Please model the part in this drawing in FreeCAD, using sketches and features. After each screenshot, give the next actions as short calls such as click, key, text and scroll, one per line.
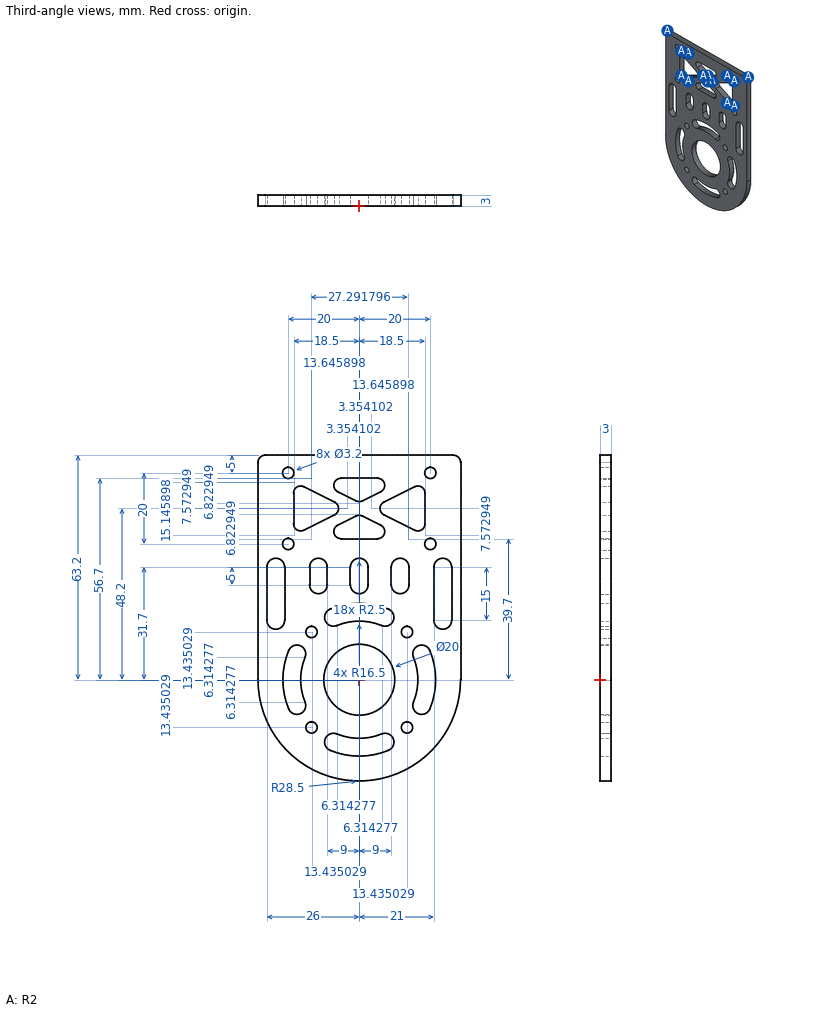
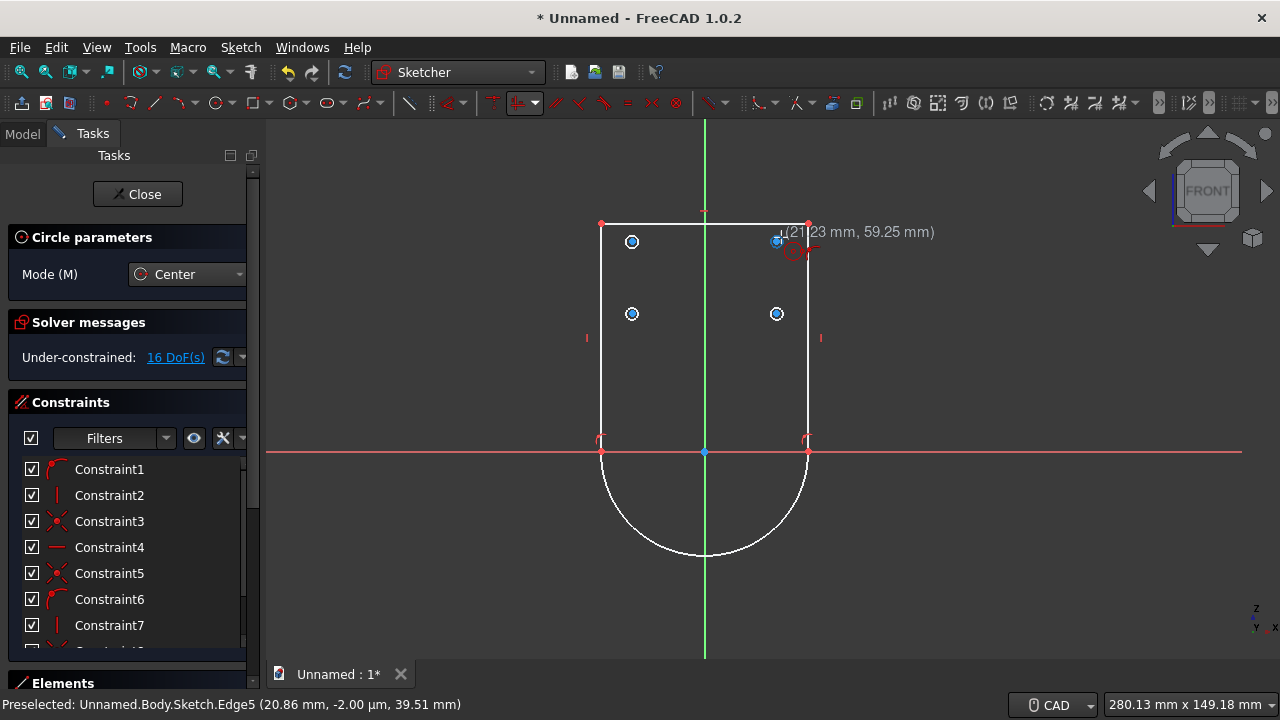
scroll(656, 403, up, 7)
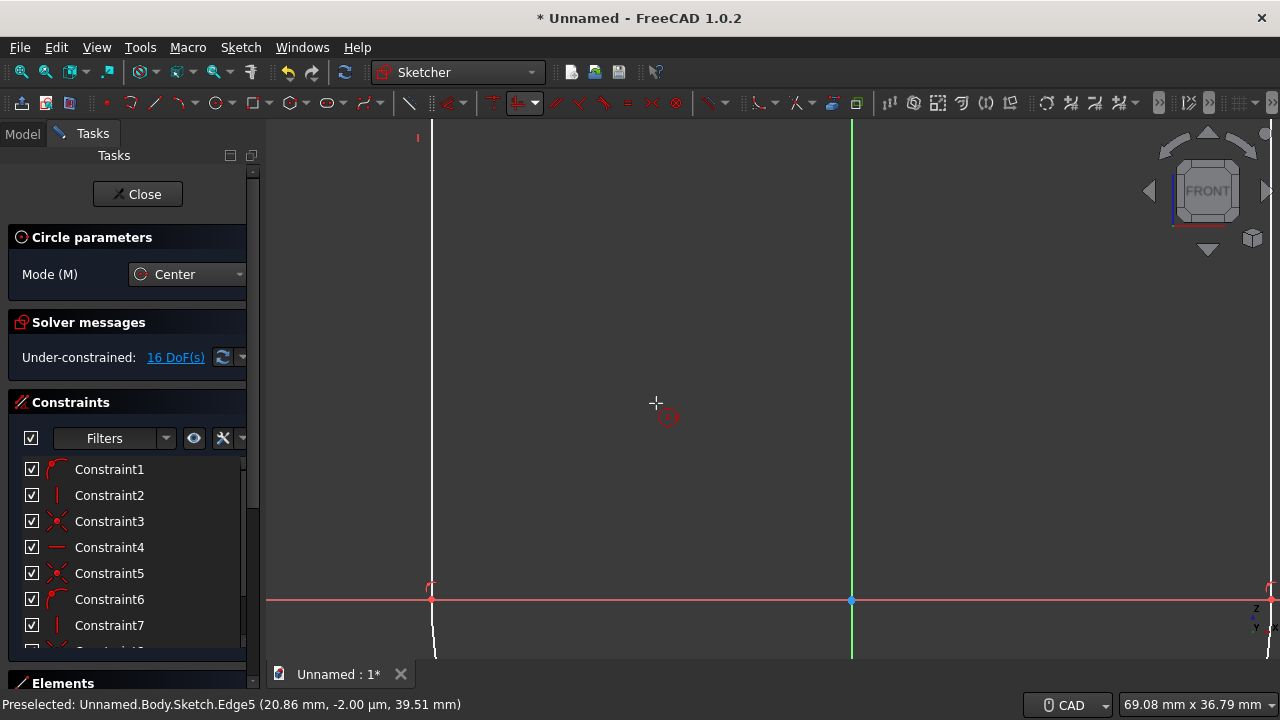
scroll(656, 403, down, 7)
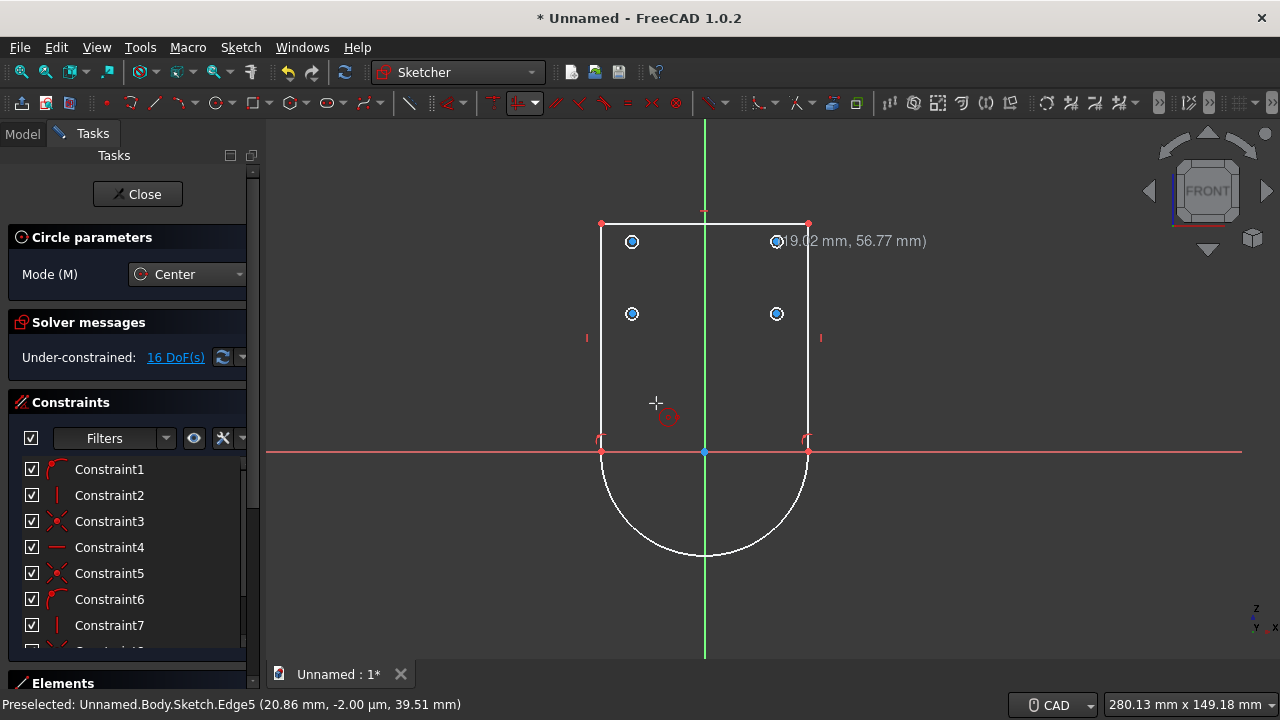
click(656, 403)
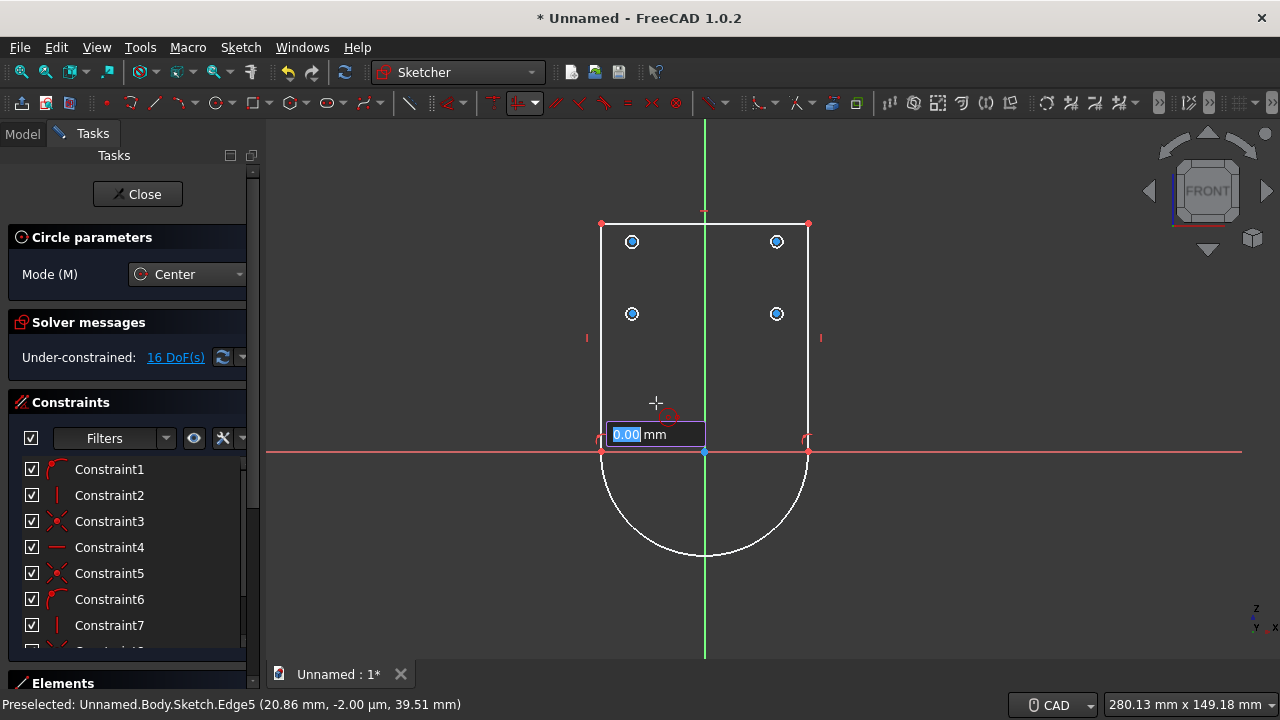
scroll(660, 399, up, 6)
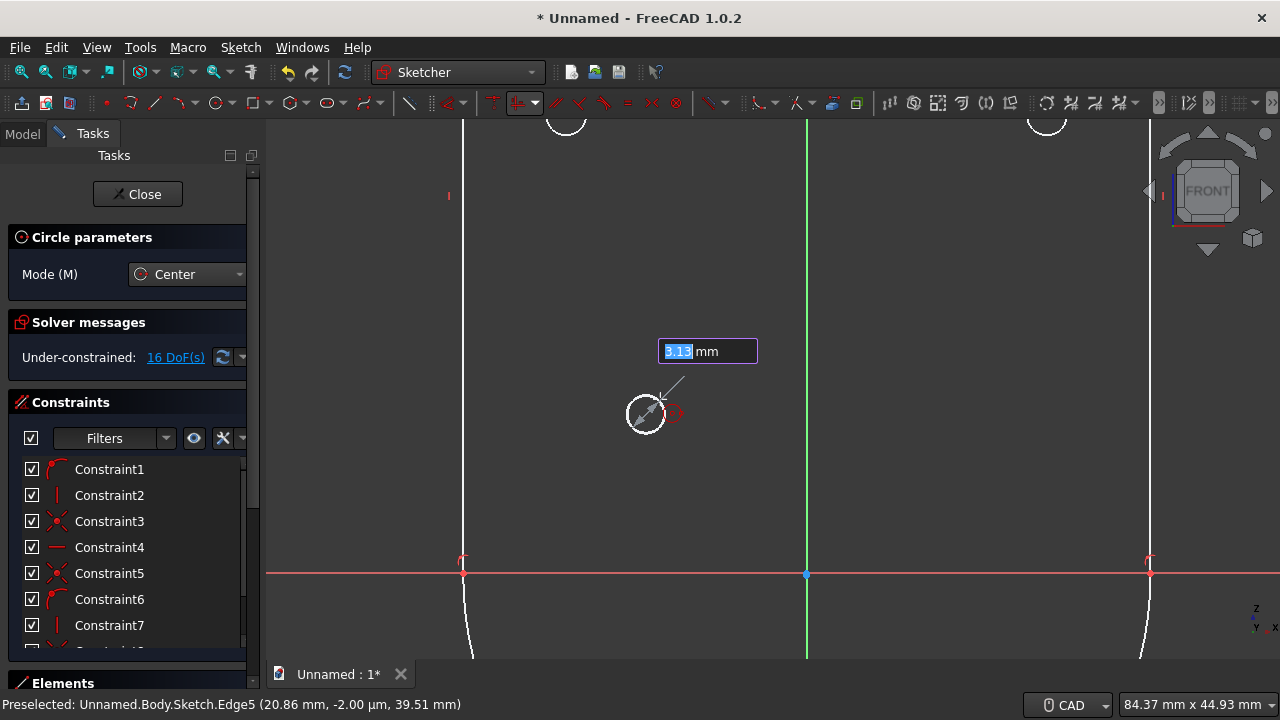
click(659, 398)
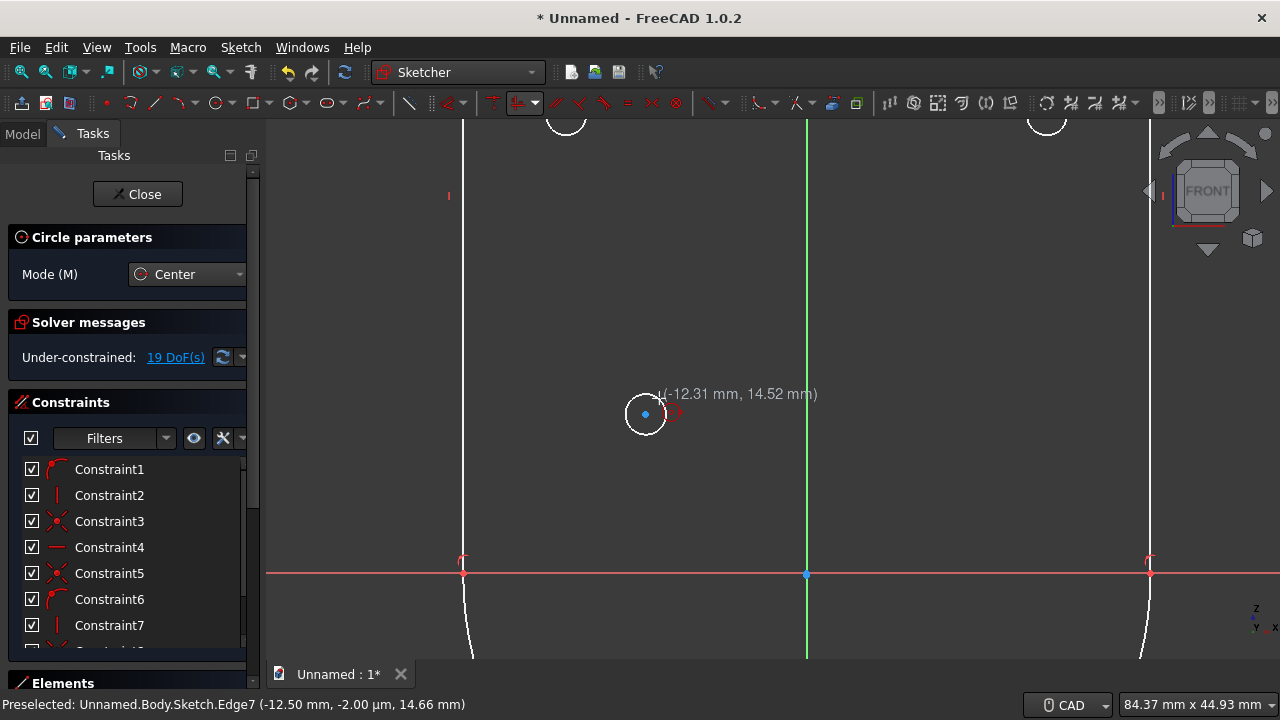
scroll(660, 399, down, 6)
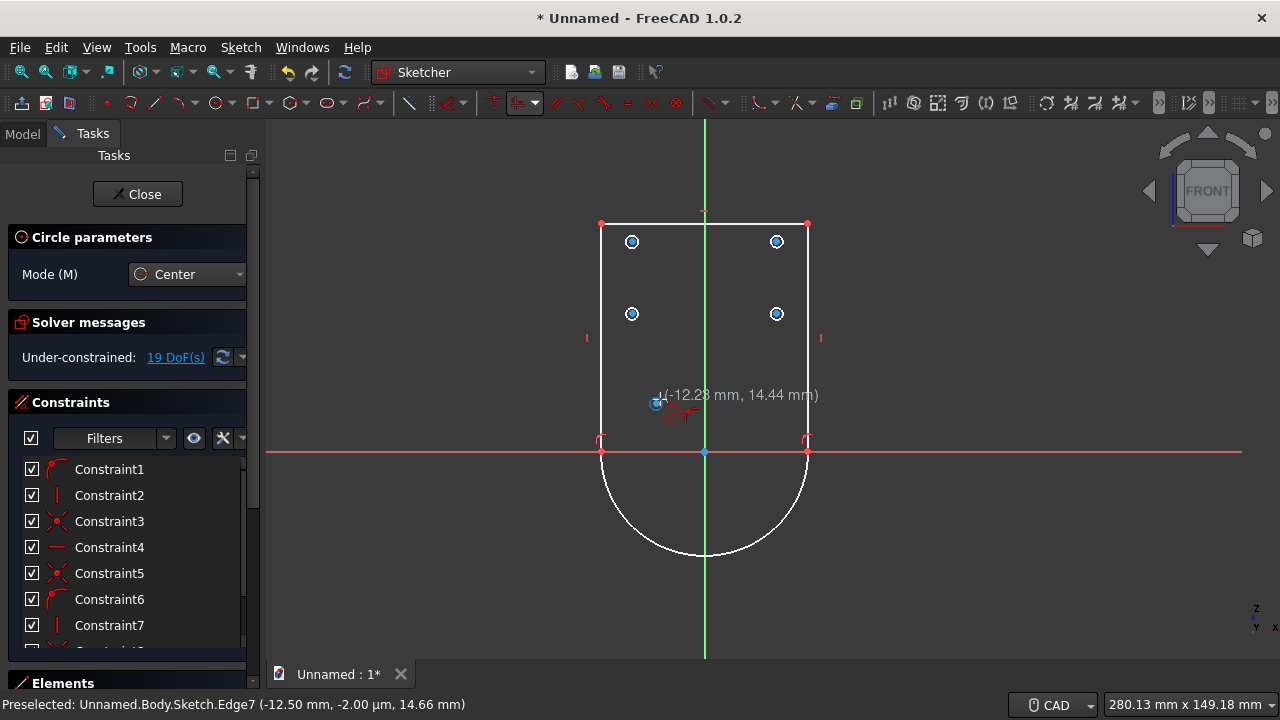
scroll(656, 501, up, 7)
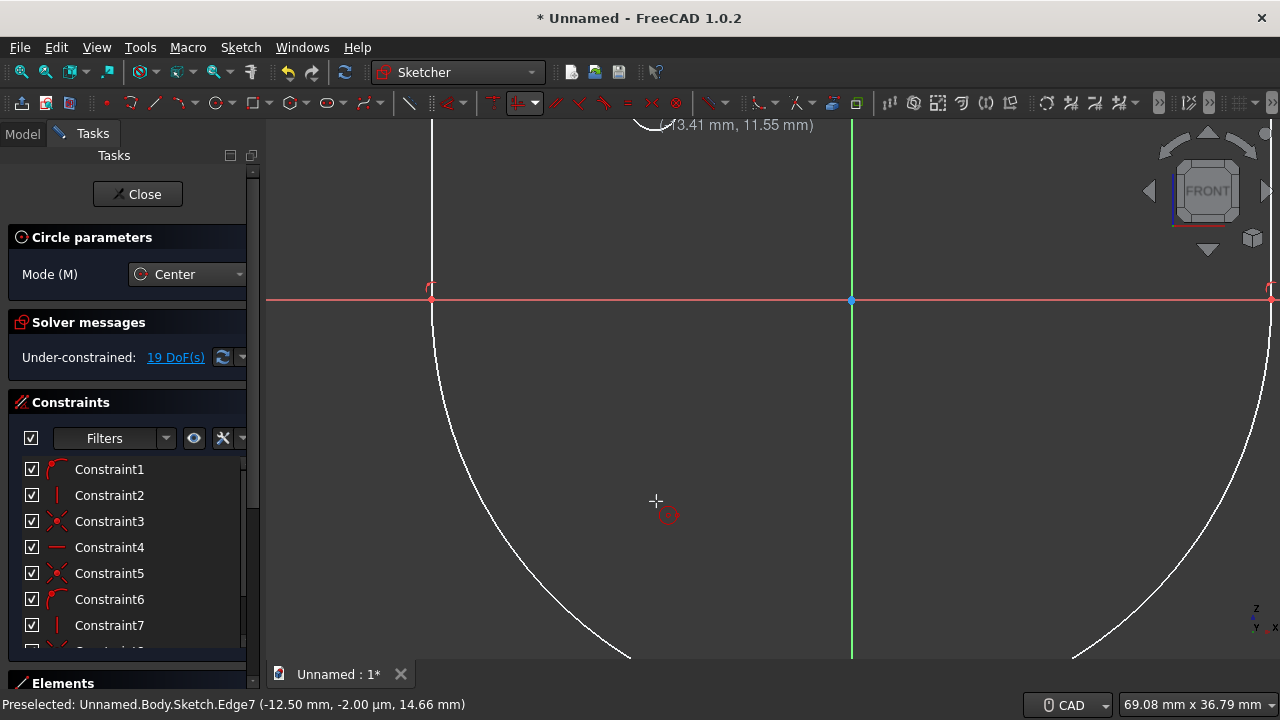
scroll(656, 502, down, 7)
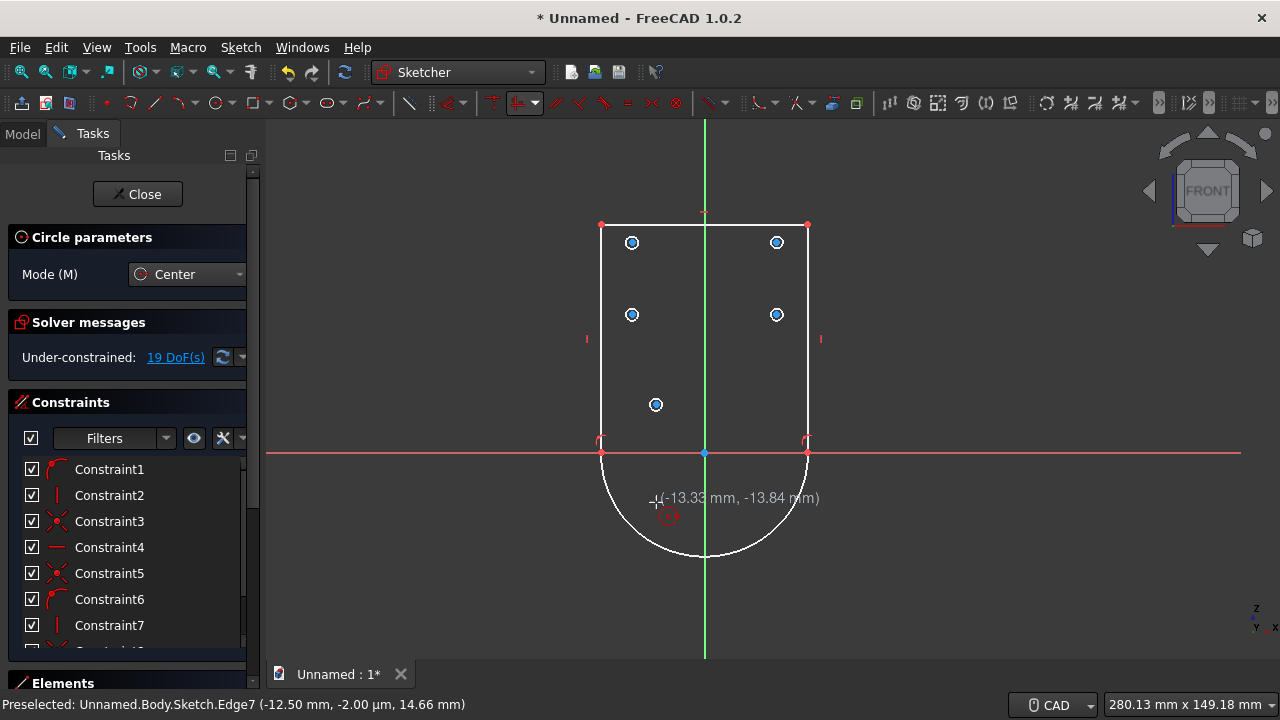
click(656, 501)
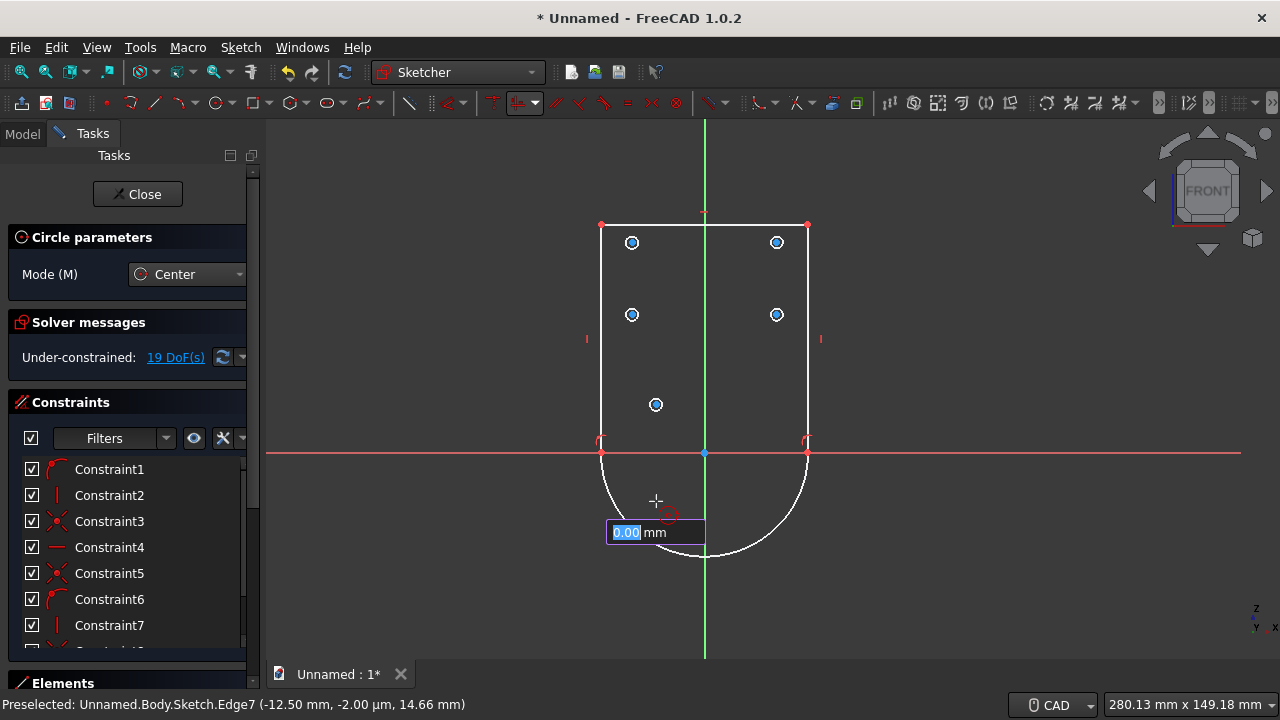
scroll(660, 497, up, 6)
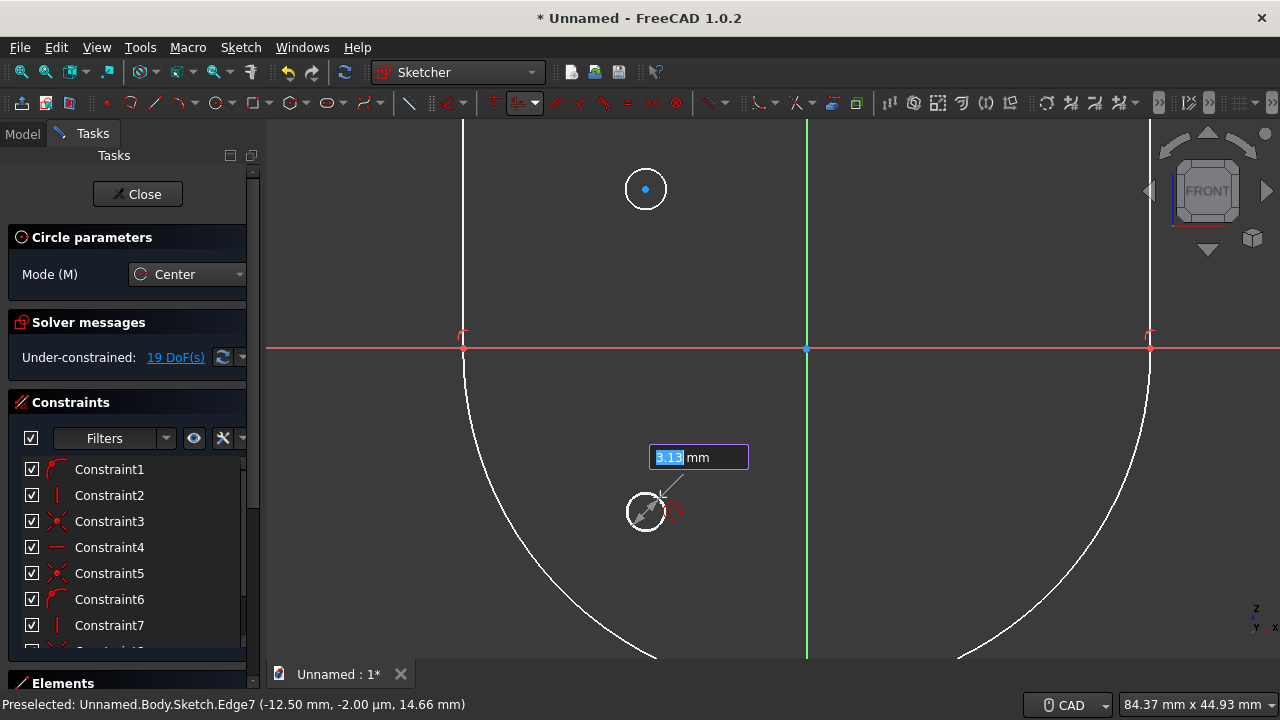
click(659, 496)